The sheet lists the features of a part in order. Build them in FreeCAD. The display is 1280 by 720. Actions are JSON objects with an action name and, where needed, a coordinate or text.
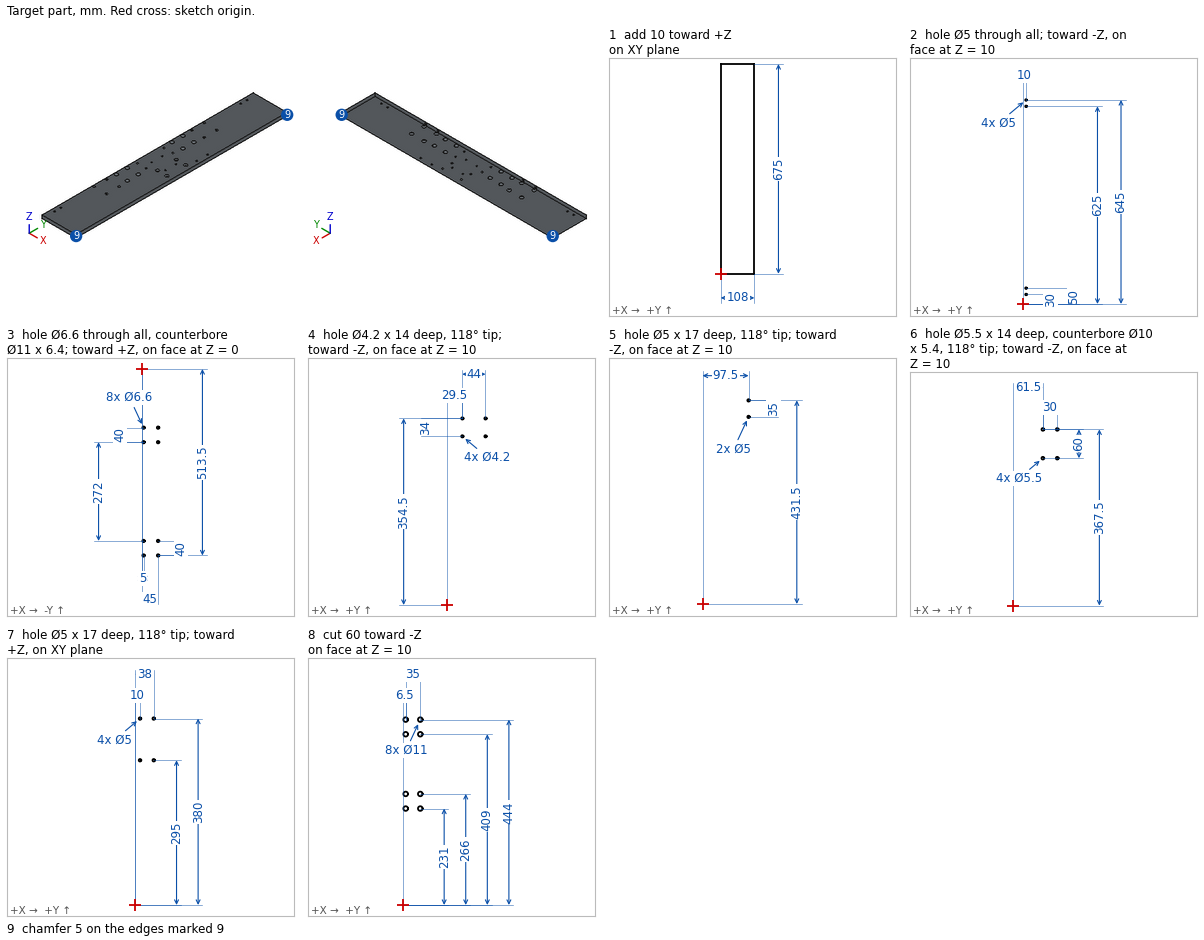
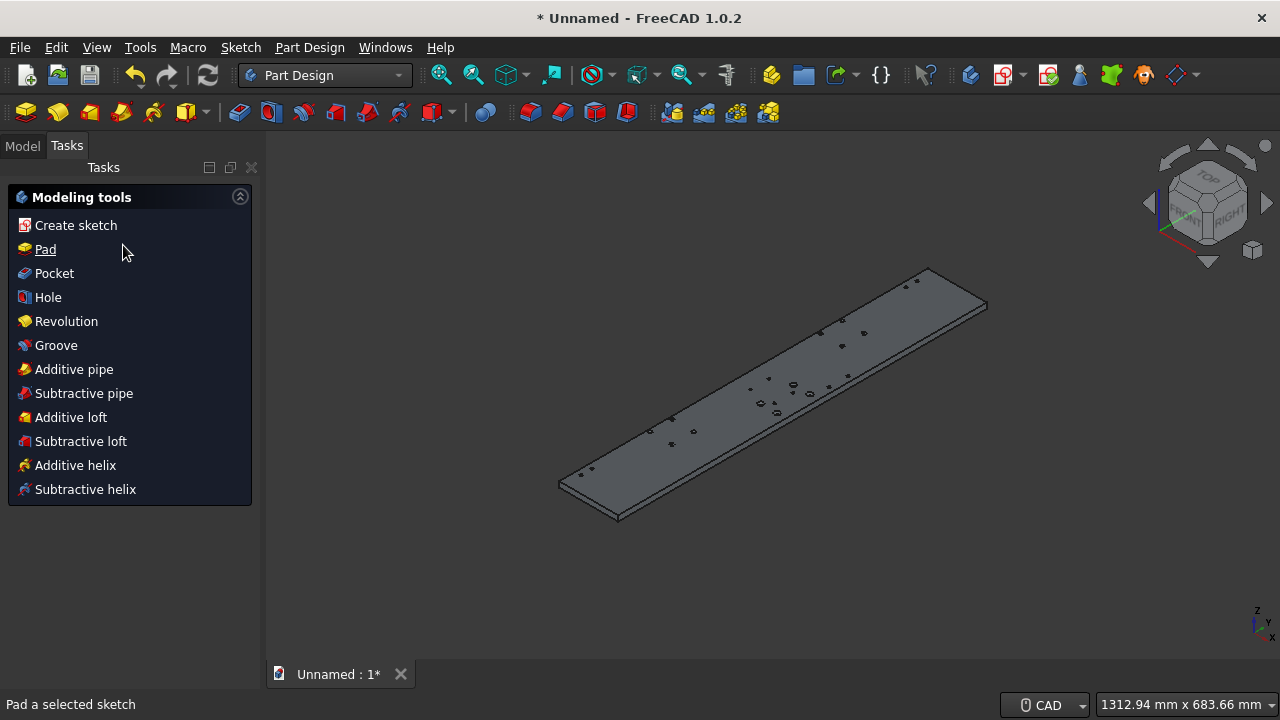
{"action": "left_click", "coordinate": [272, 112]}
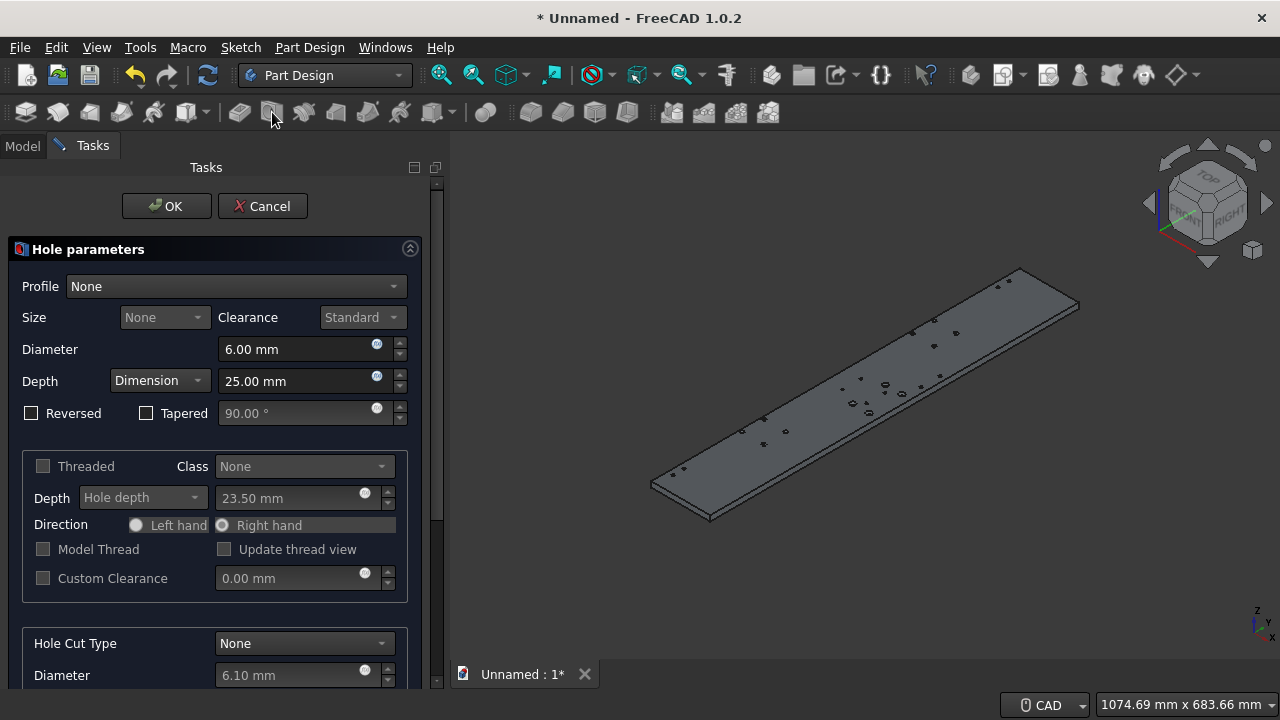
{"action": "triple_click", "coordinate": [305, 349]}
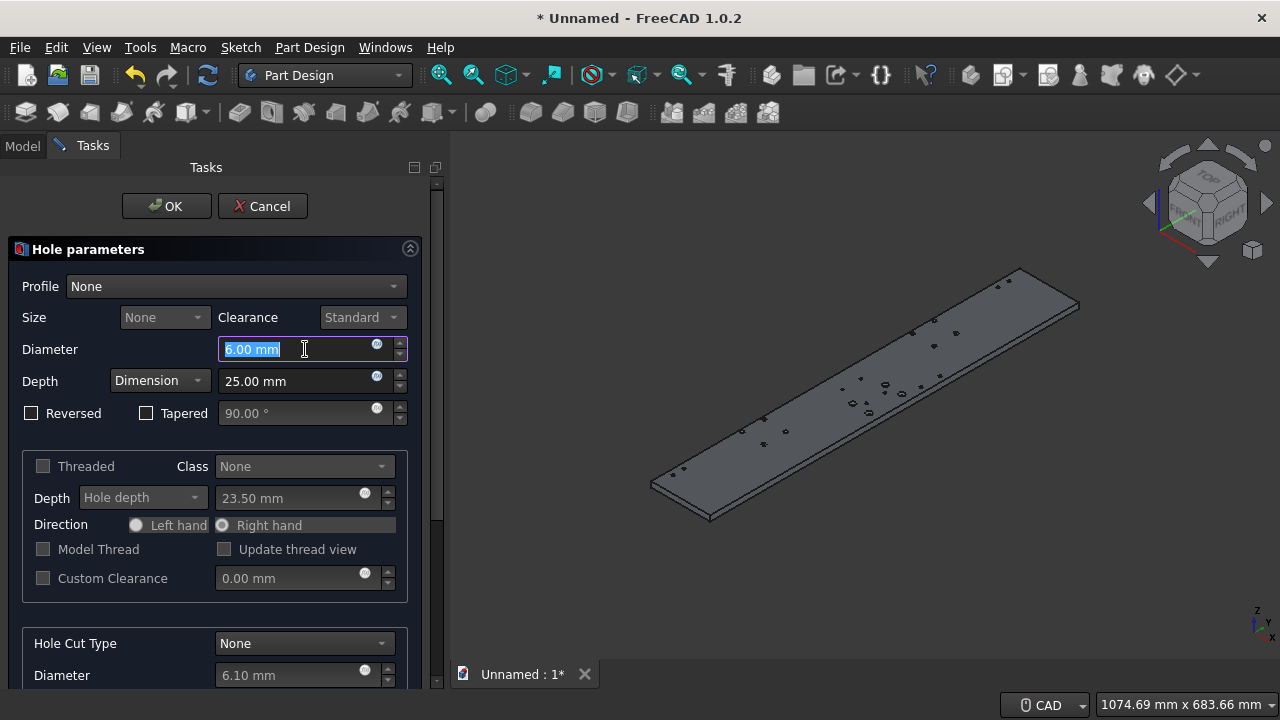
{"action": "type", "text": "5"}
{"action": "key", "text": "Tab"}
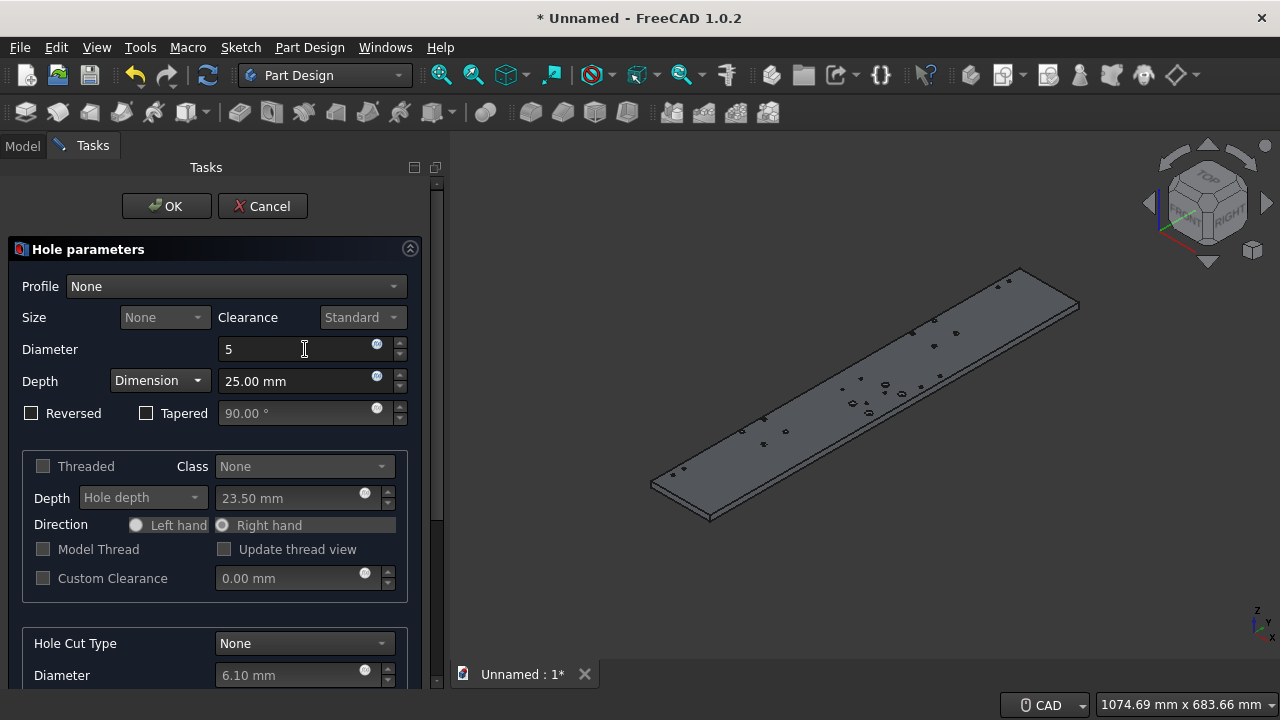
{"action": "triple_click", "coordinate": [305, 381]}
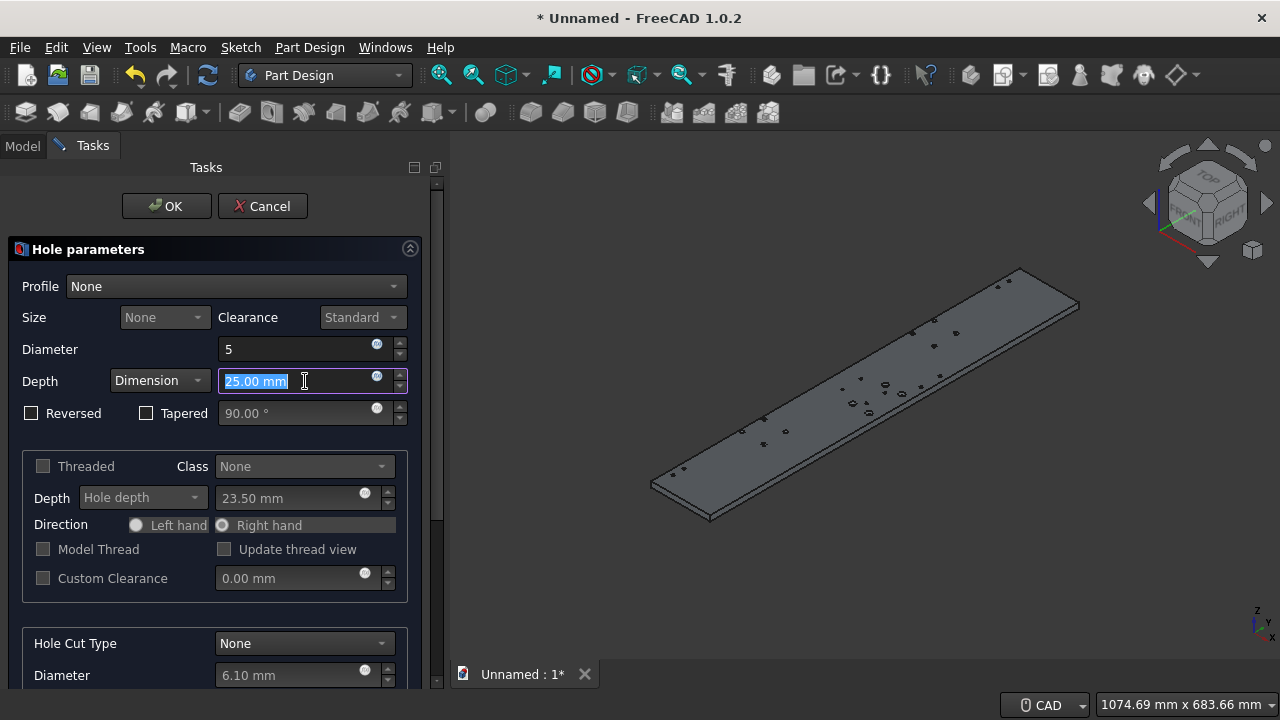
{"action": "type", "text": "17"}
{"action": "key", "text": "Tab"}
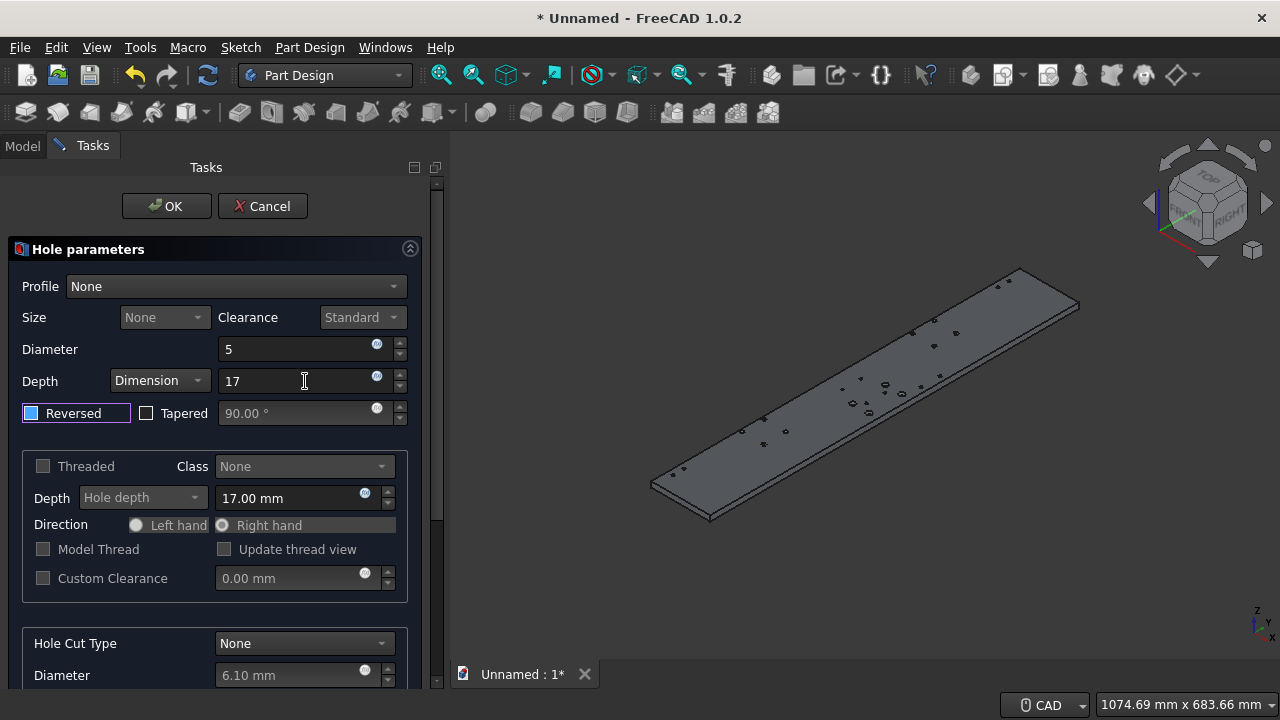
{"action": "left_click", "coordinate": [30, 413]}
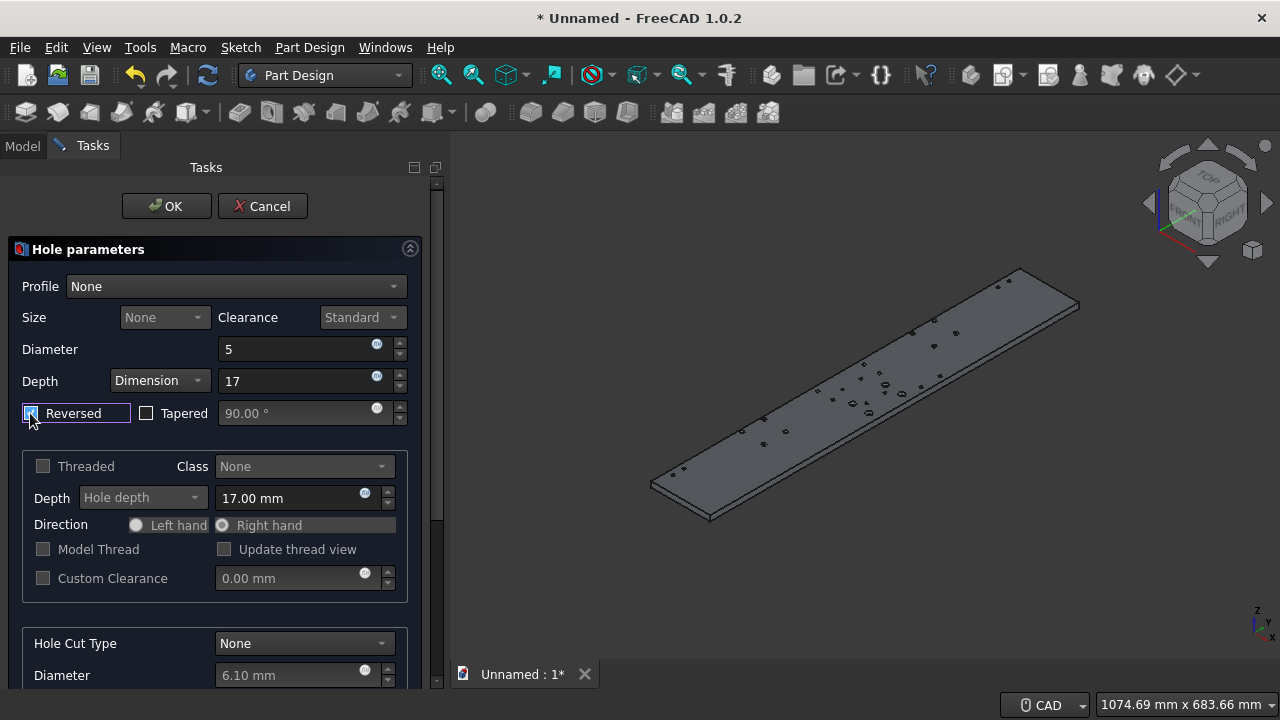
{"action": "left_click", "coordinate": [167, 206]}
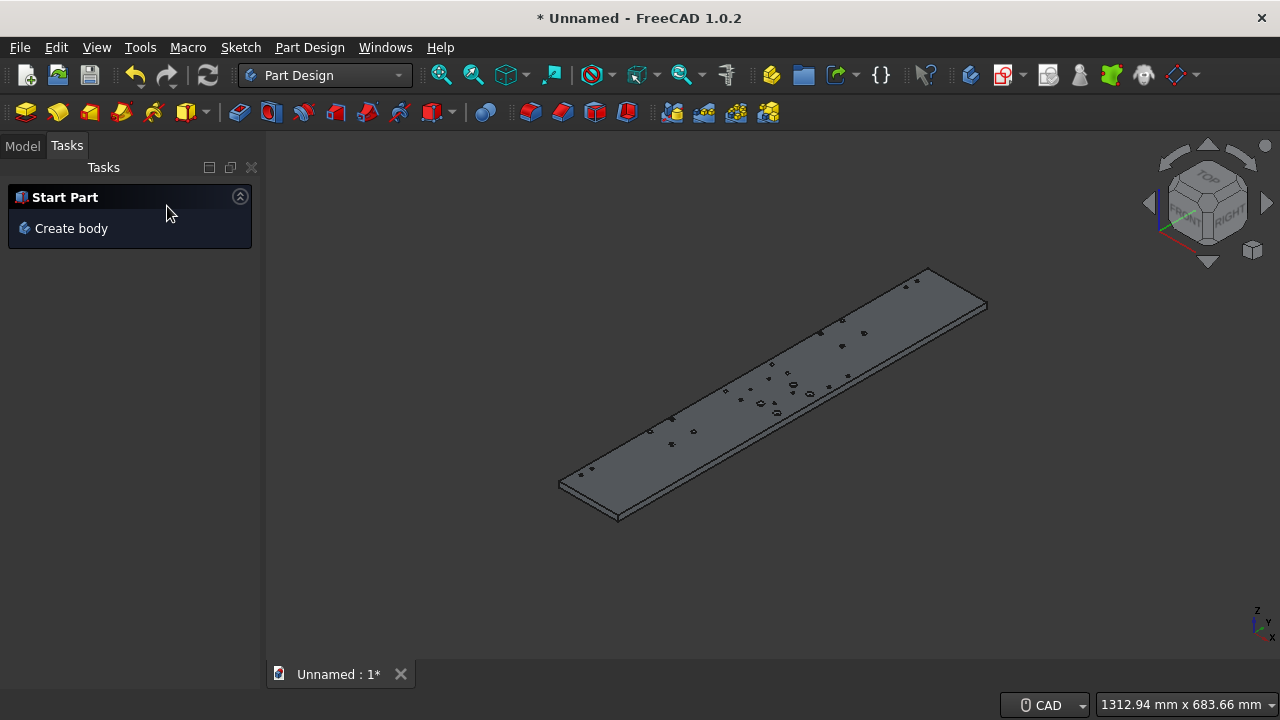
{"action": "left_click", "coordinate": [931, 300]}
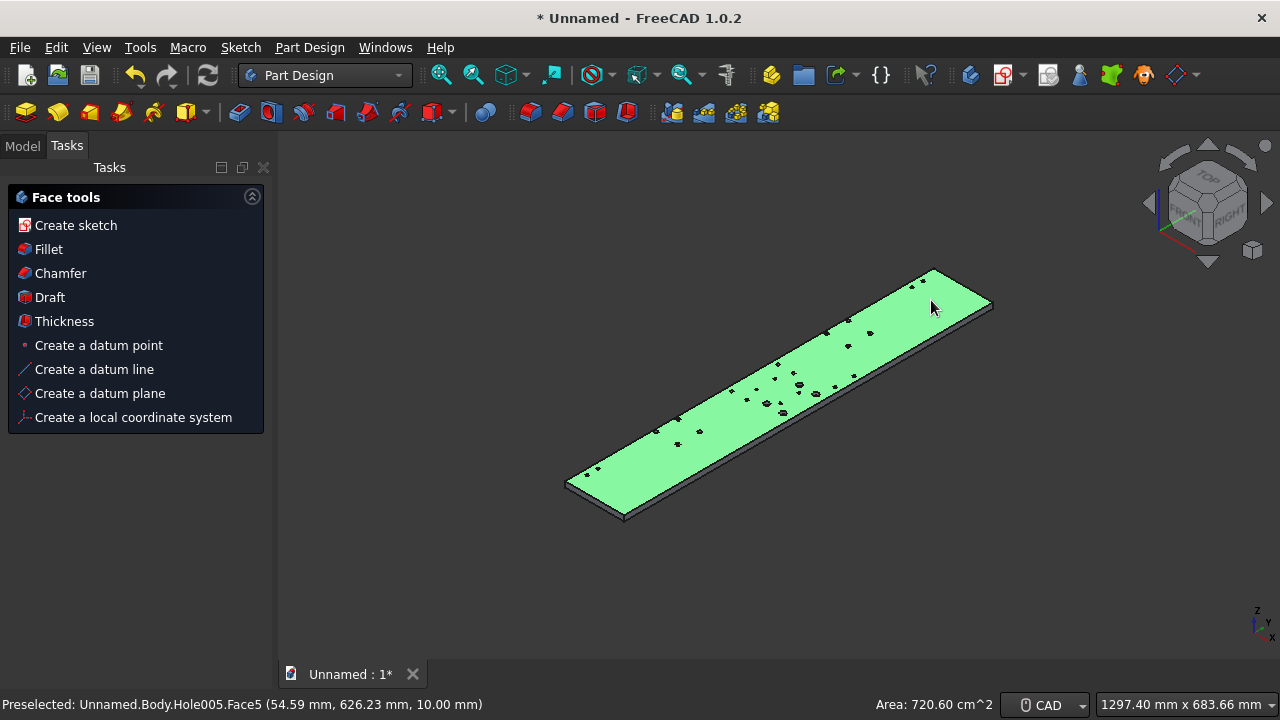
{"action": "left_click", "coordinate": [1004, 76]}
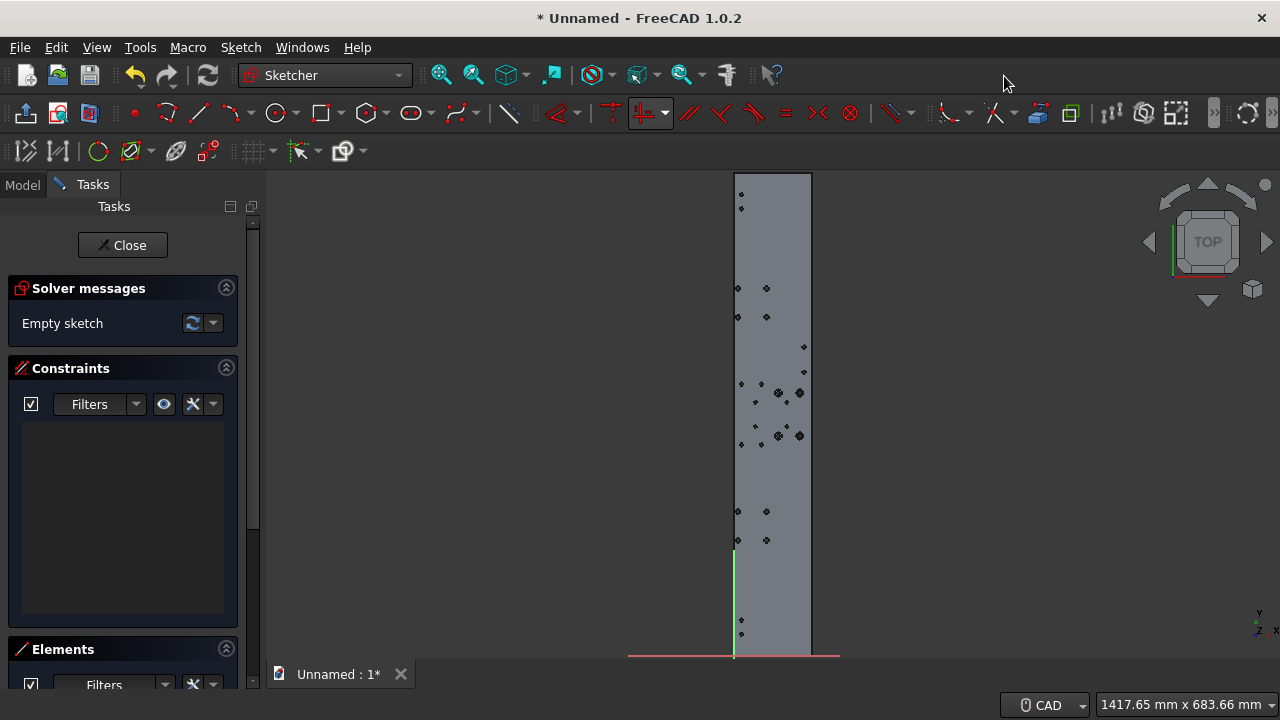
{"action": "scroll", "coordinate": [494, 198], "scroll_direction": "down", "scroll_amount": 1}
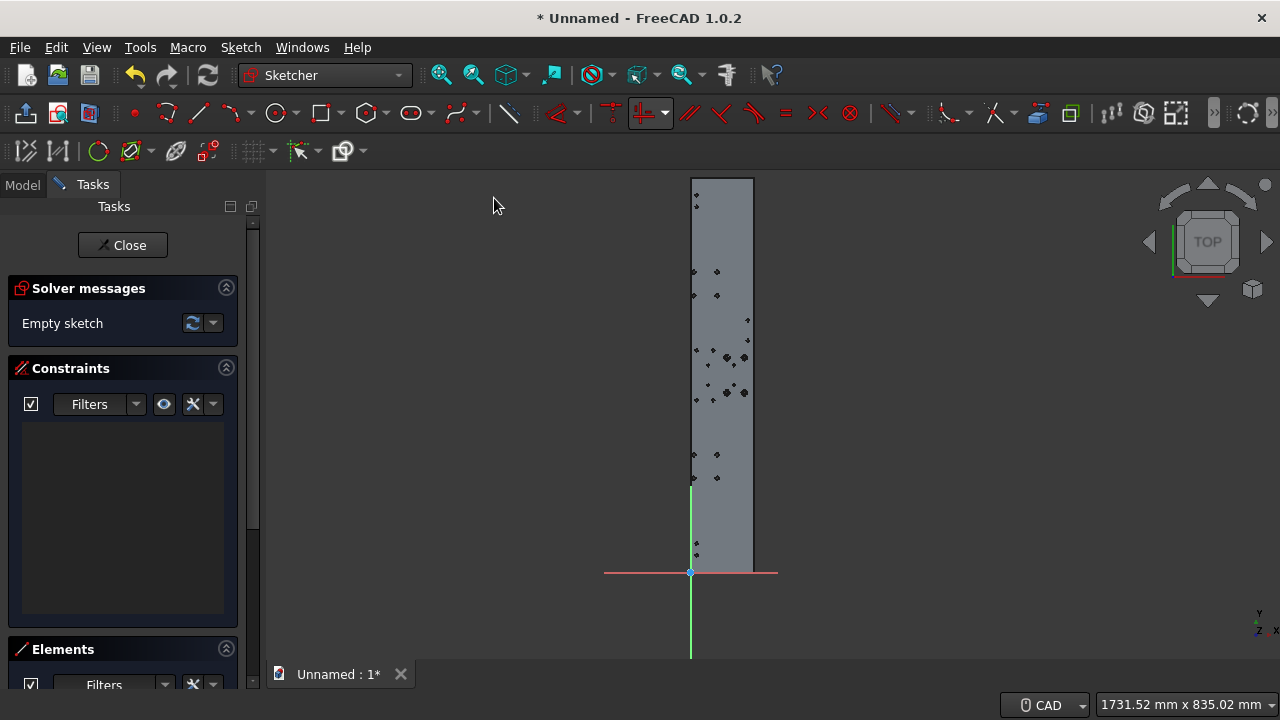
{"action": "left_click", "coordinate": [276, 114]}